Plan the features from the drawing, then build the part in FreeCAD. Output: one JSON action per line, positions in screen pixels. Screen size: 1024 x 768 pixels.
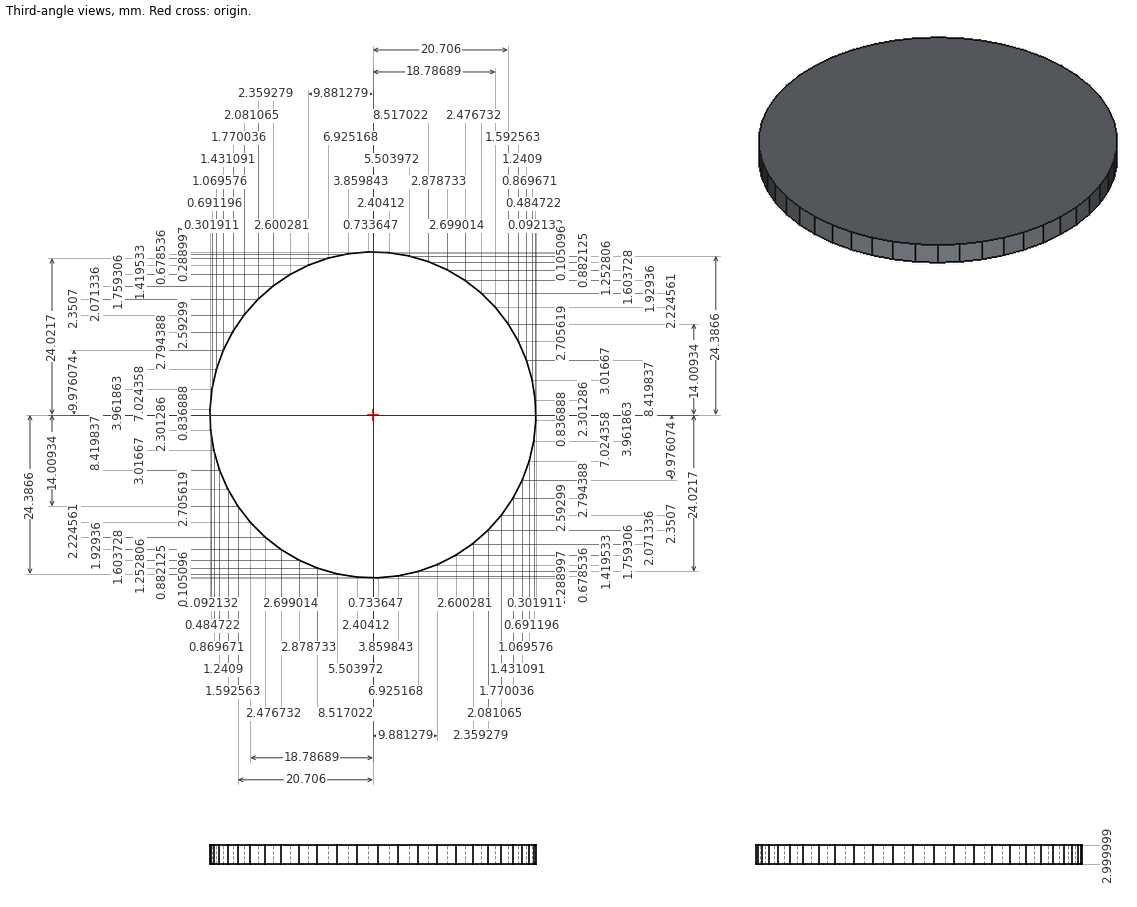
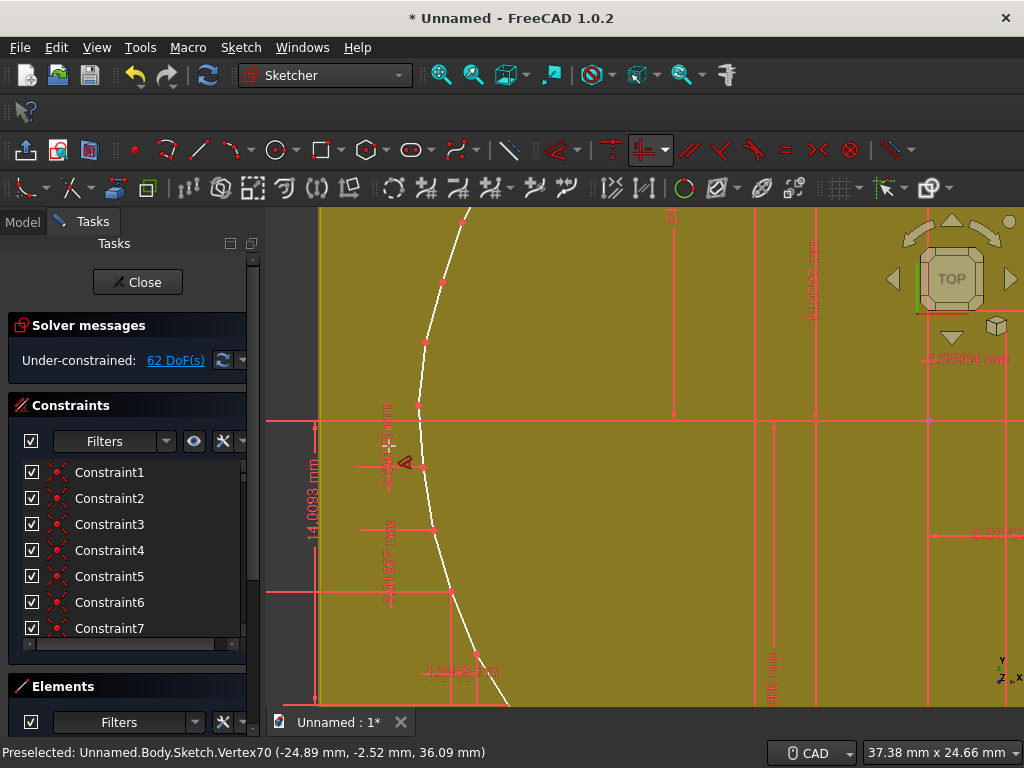
{"action": "scroll", "coordinate": [419, 405], "scroll_direction": "up", "scroll_amount": 5}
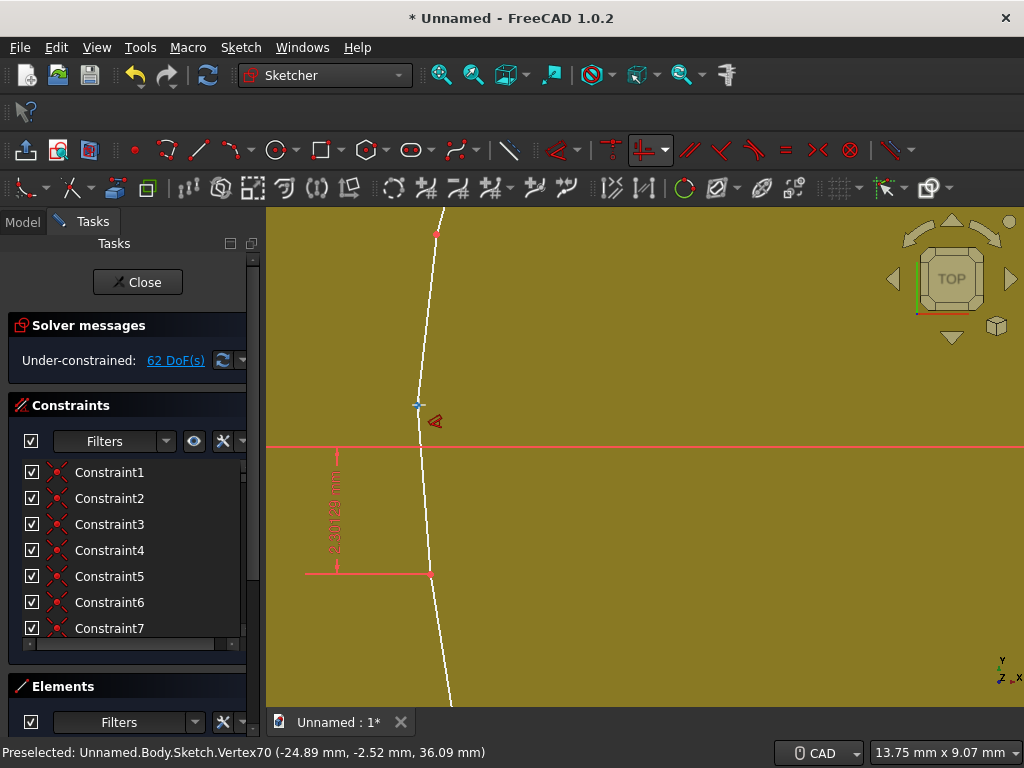
{"action": "left_click", "coordinate": [417, 405]}
{"action": "left_click", "coordinate": [383, 426]}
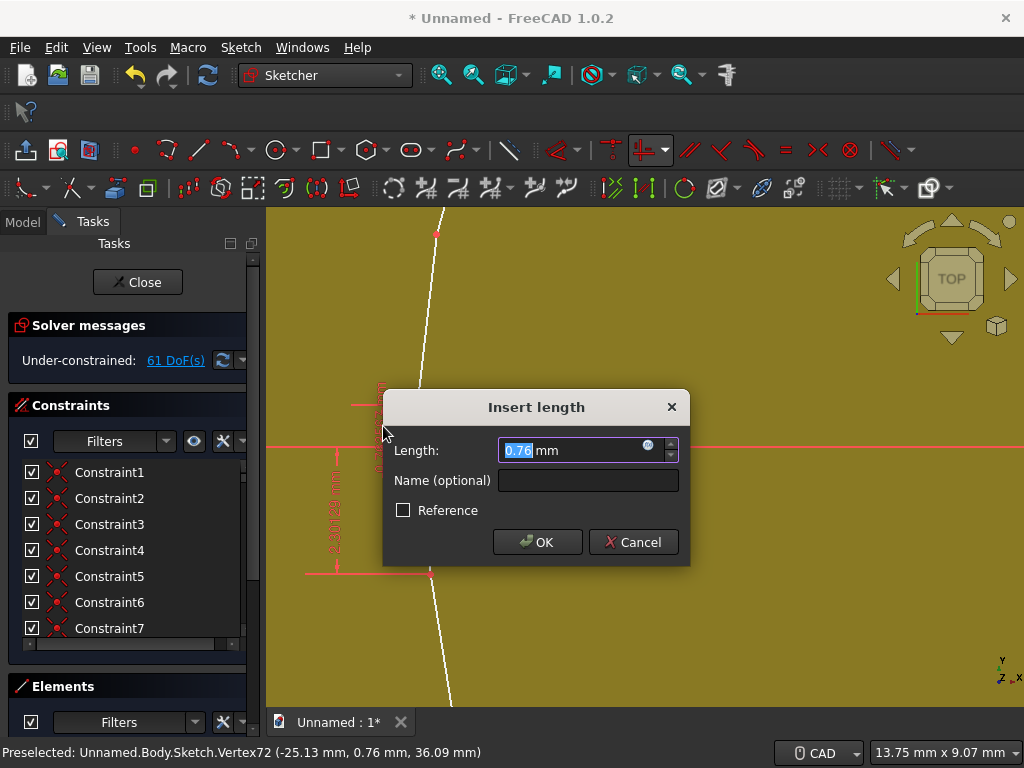
{"action": "type", "text": "0.836888"}
{"action": "key", "text": "Return"}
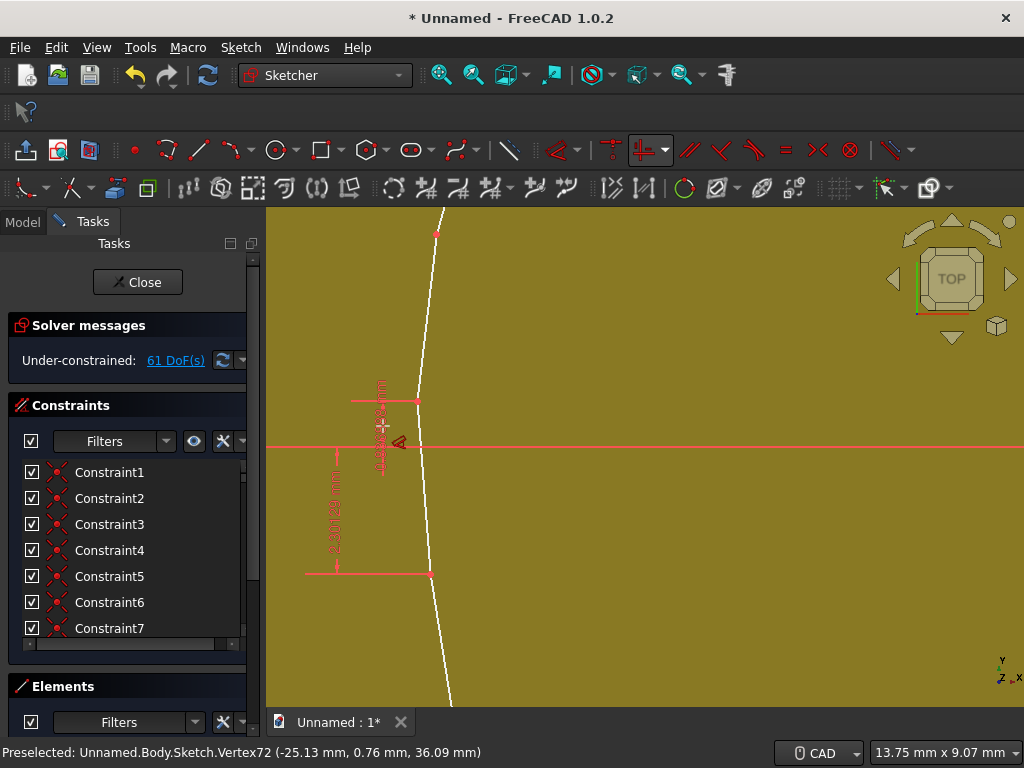
{"action": "scroll", "coordinate": [424, 458], "scroll_direction": "down", "scroll_amount": 11}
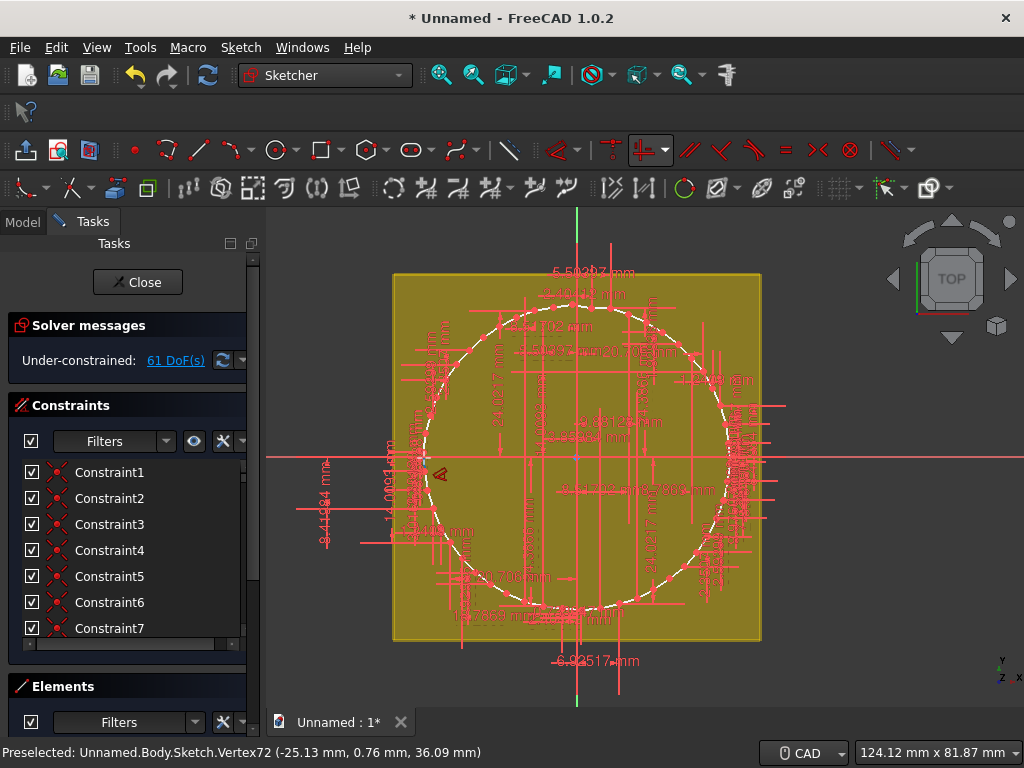
{"action": "scroll", "coordinate": [426, 434], "scroll_direction": "up", "scroll_amount": 3}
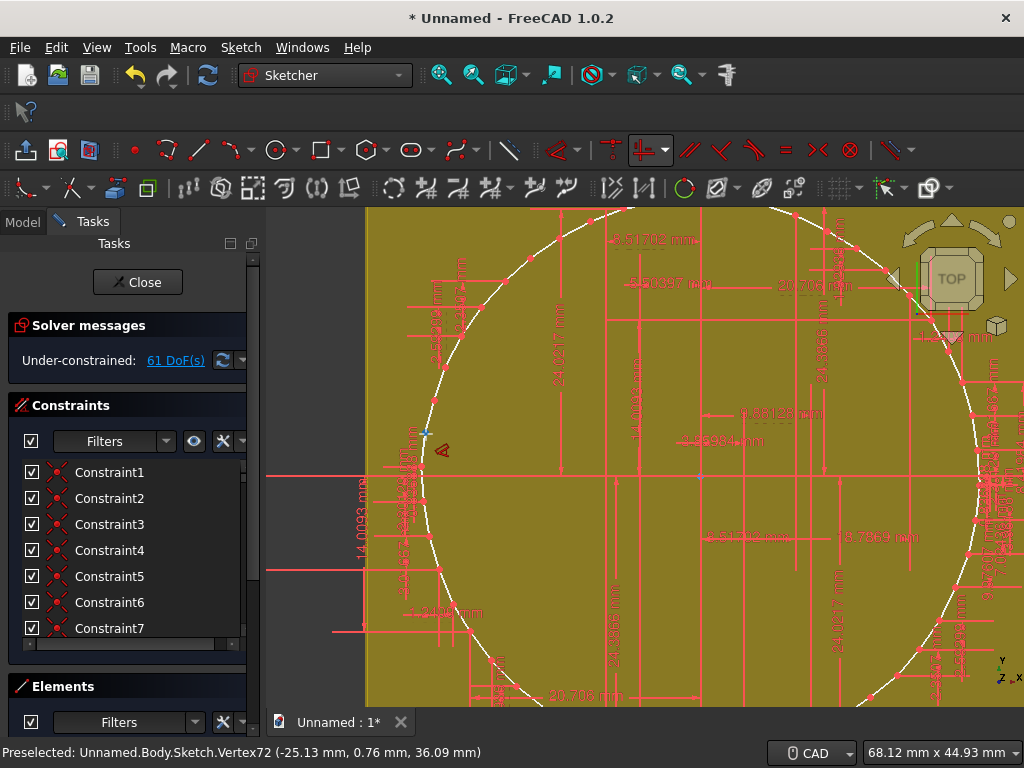
{"action": "left_click", "coordinate": [425, 433]}
{"action": "left_click", "coordinate": [391, 445]}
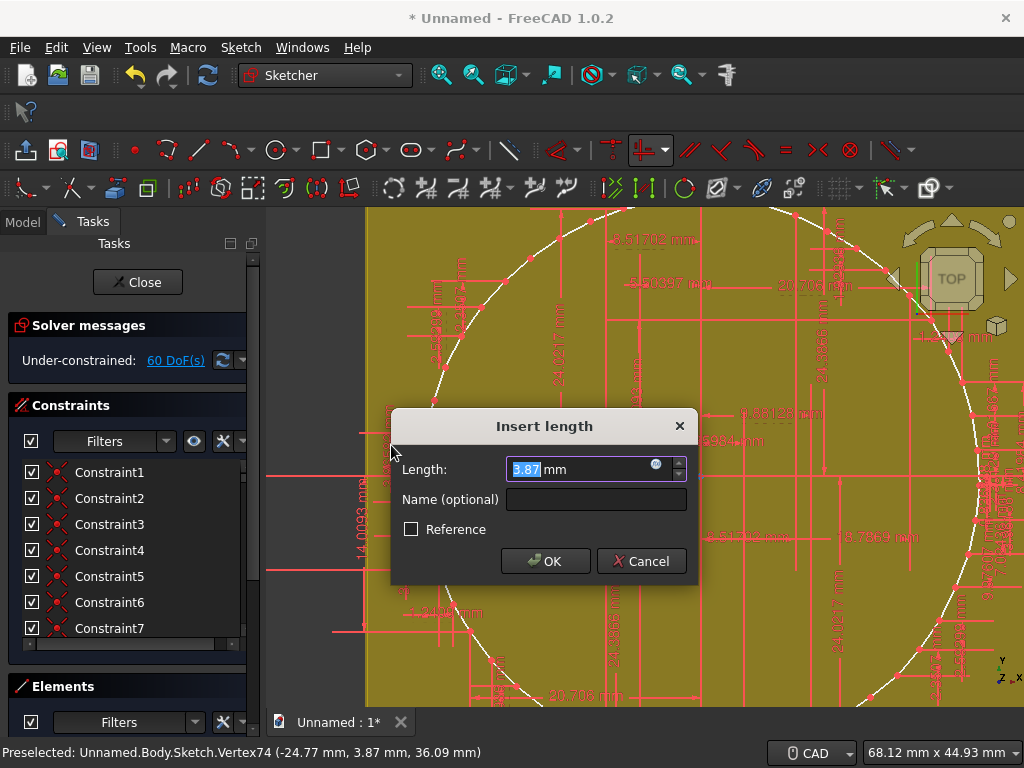
{"action": "type", "text": "3.961863"}
{"action": "key", "text": "Return"}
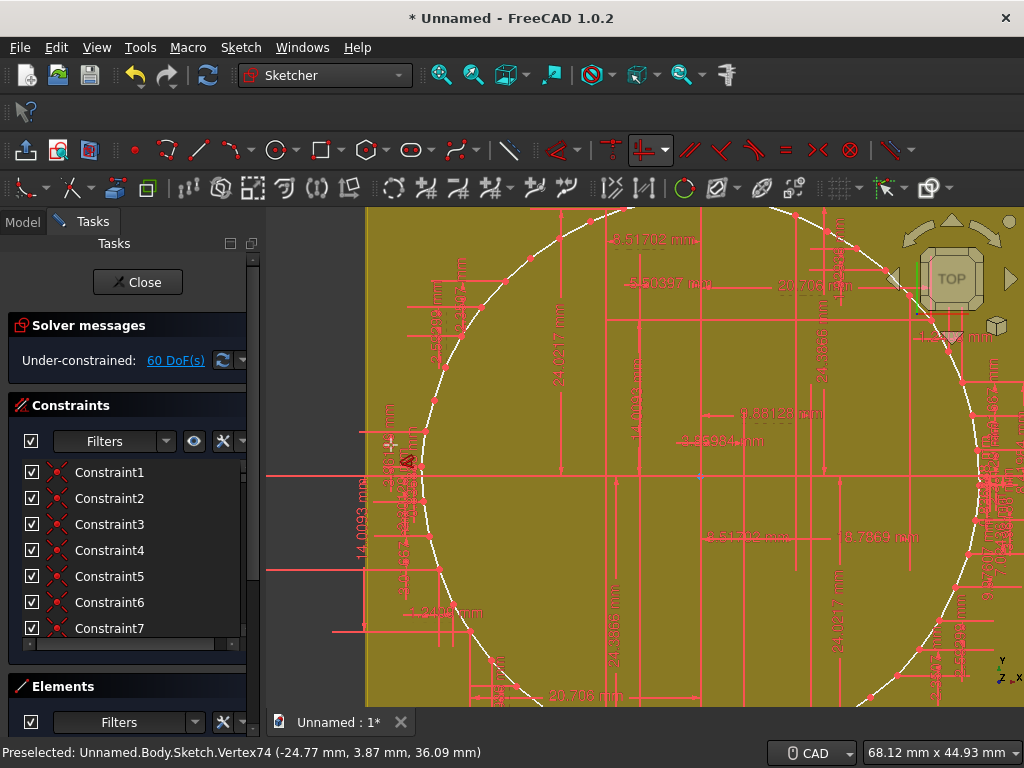
{"action": "left_click", "coordinate": [434, 400]}
{"action": "left_click", "coordinate": [400, 421]}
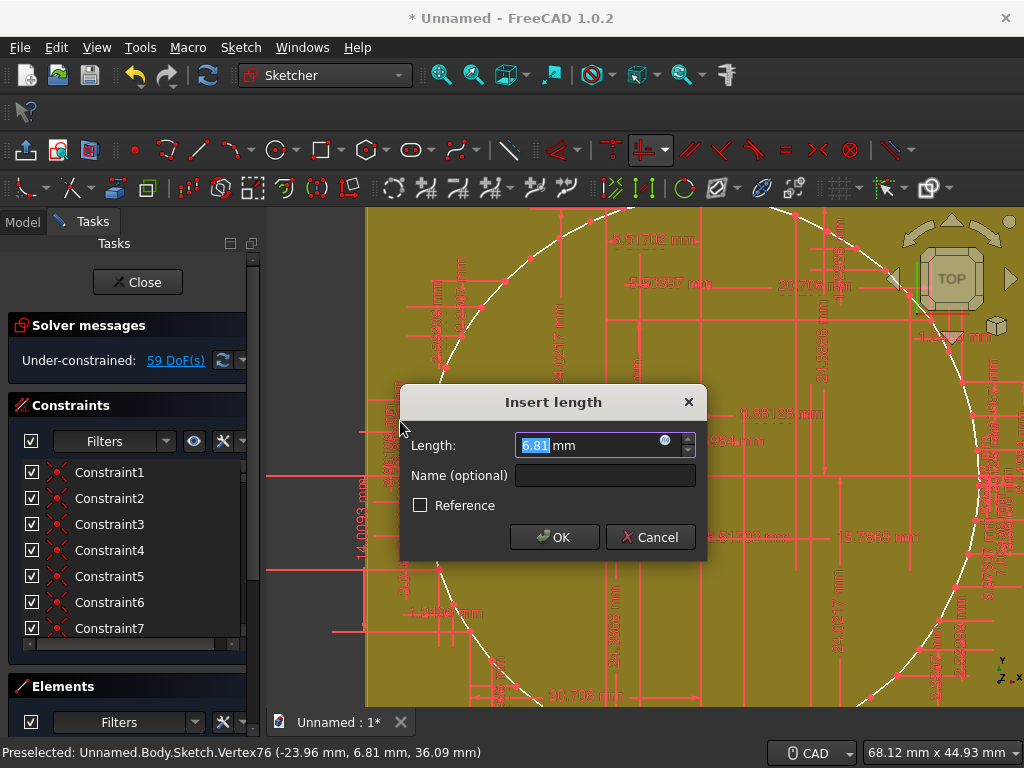
{"action": "type", "text": "7.024358"}
{"action": "key", "text": "Return"}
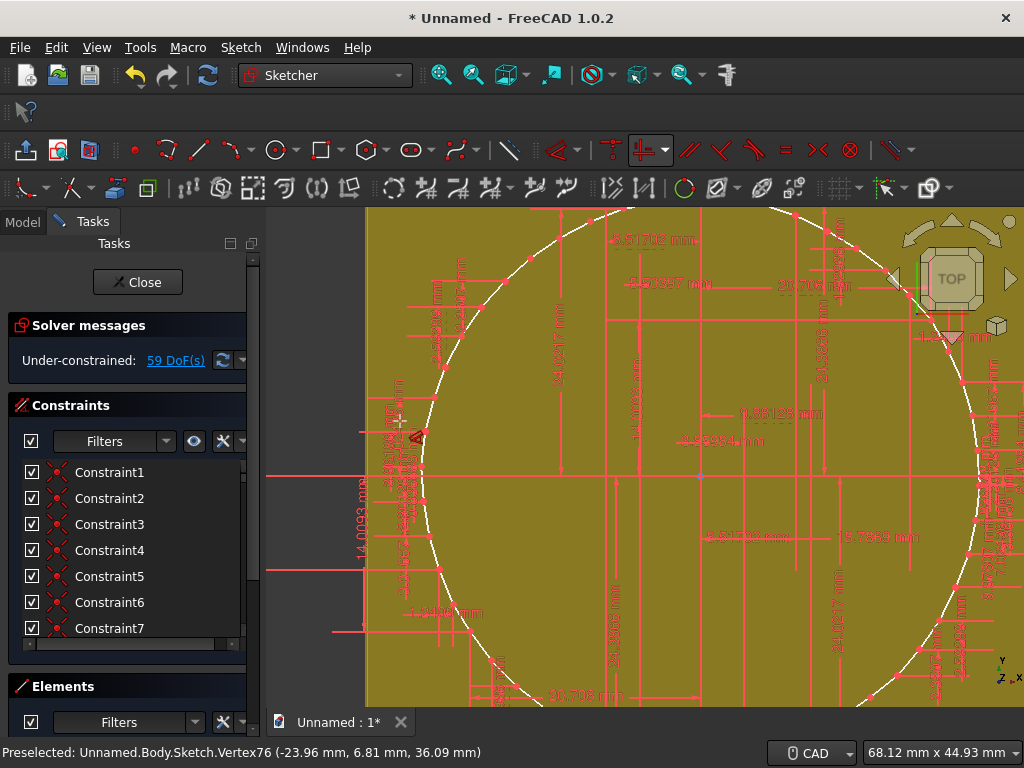
{"action": "left_click", "coordinate": [445, 367]}
{"action": "left_click", "coordinate": [411, 397]}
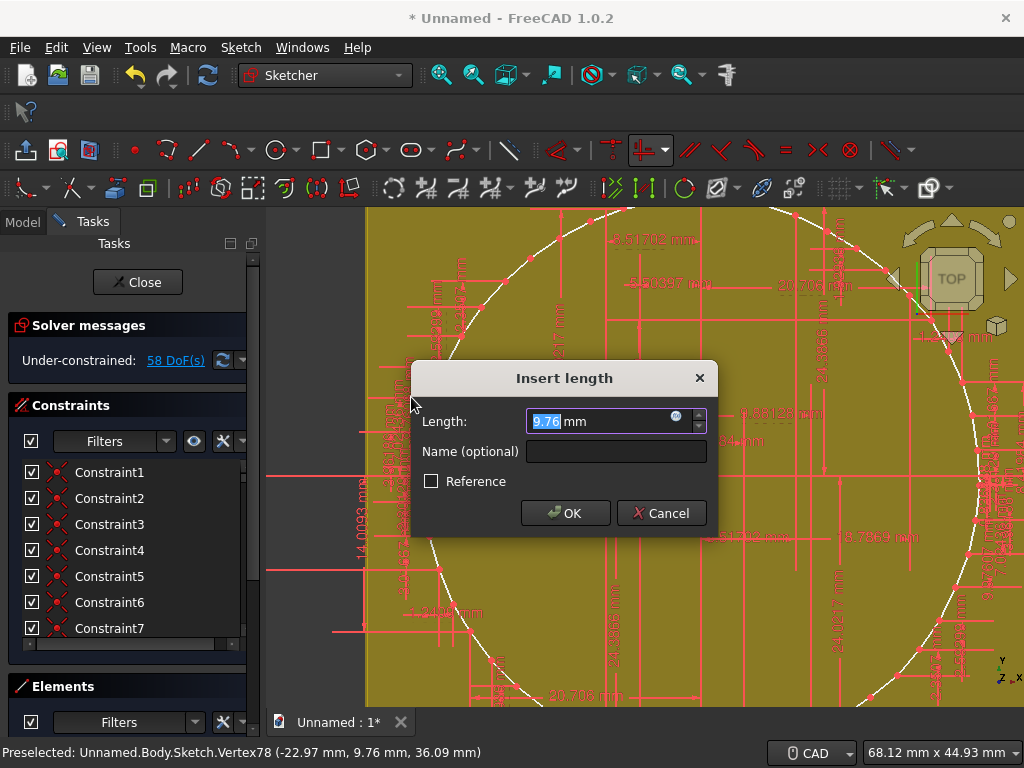
{"action": "type", "text": "9.976074"}
{"action": "key", "text": "Return"}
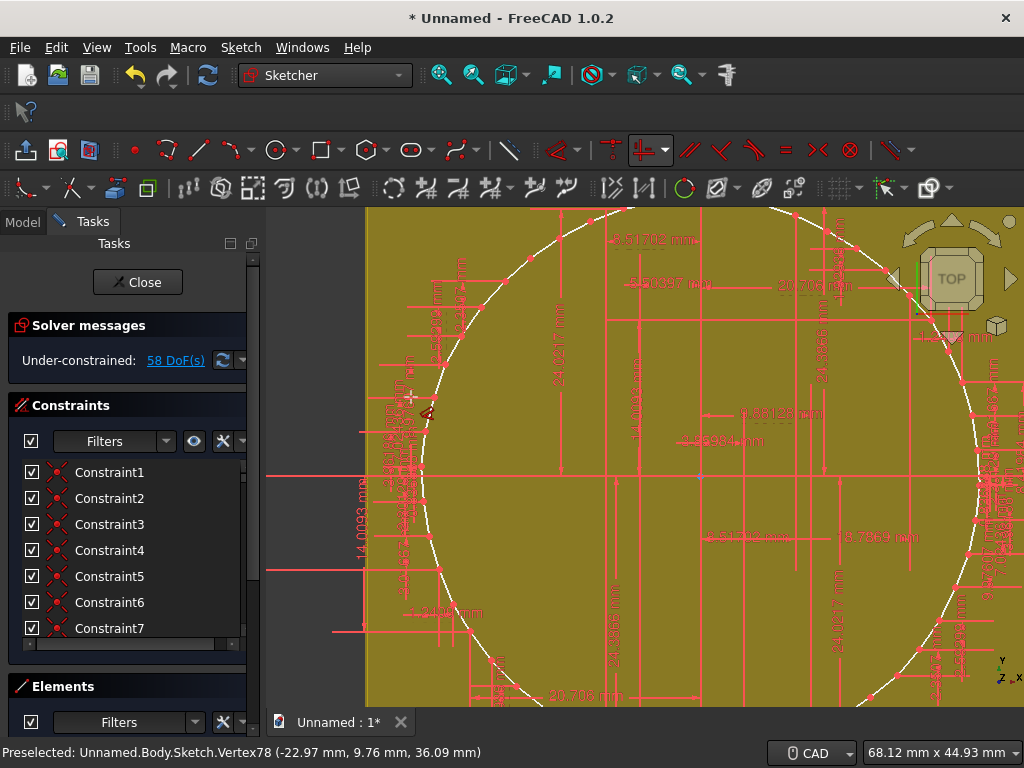
{"action": "scroll", "coordinate": [425, 434], "scroll_direction": "down", "scroll_amount": 3}